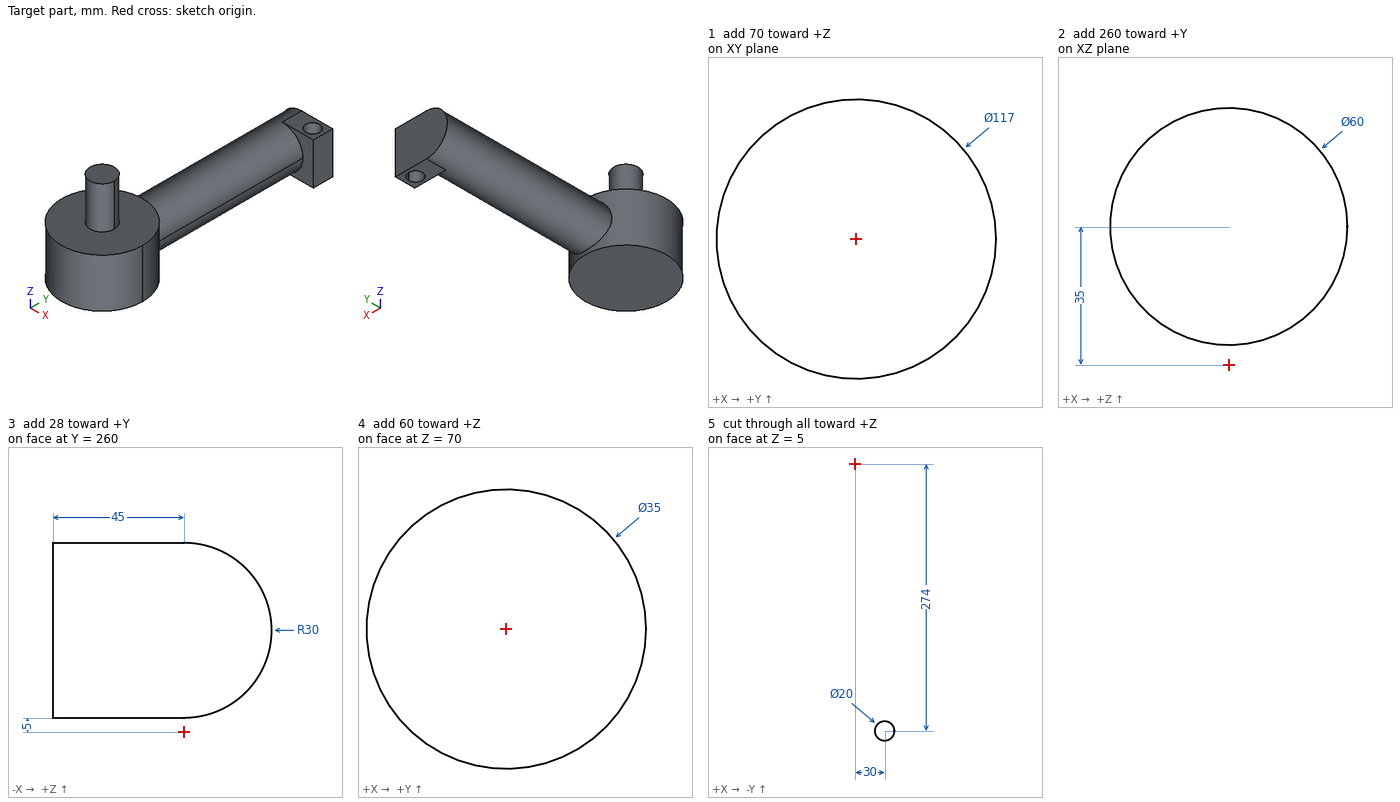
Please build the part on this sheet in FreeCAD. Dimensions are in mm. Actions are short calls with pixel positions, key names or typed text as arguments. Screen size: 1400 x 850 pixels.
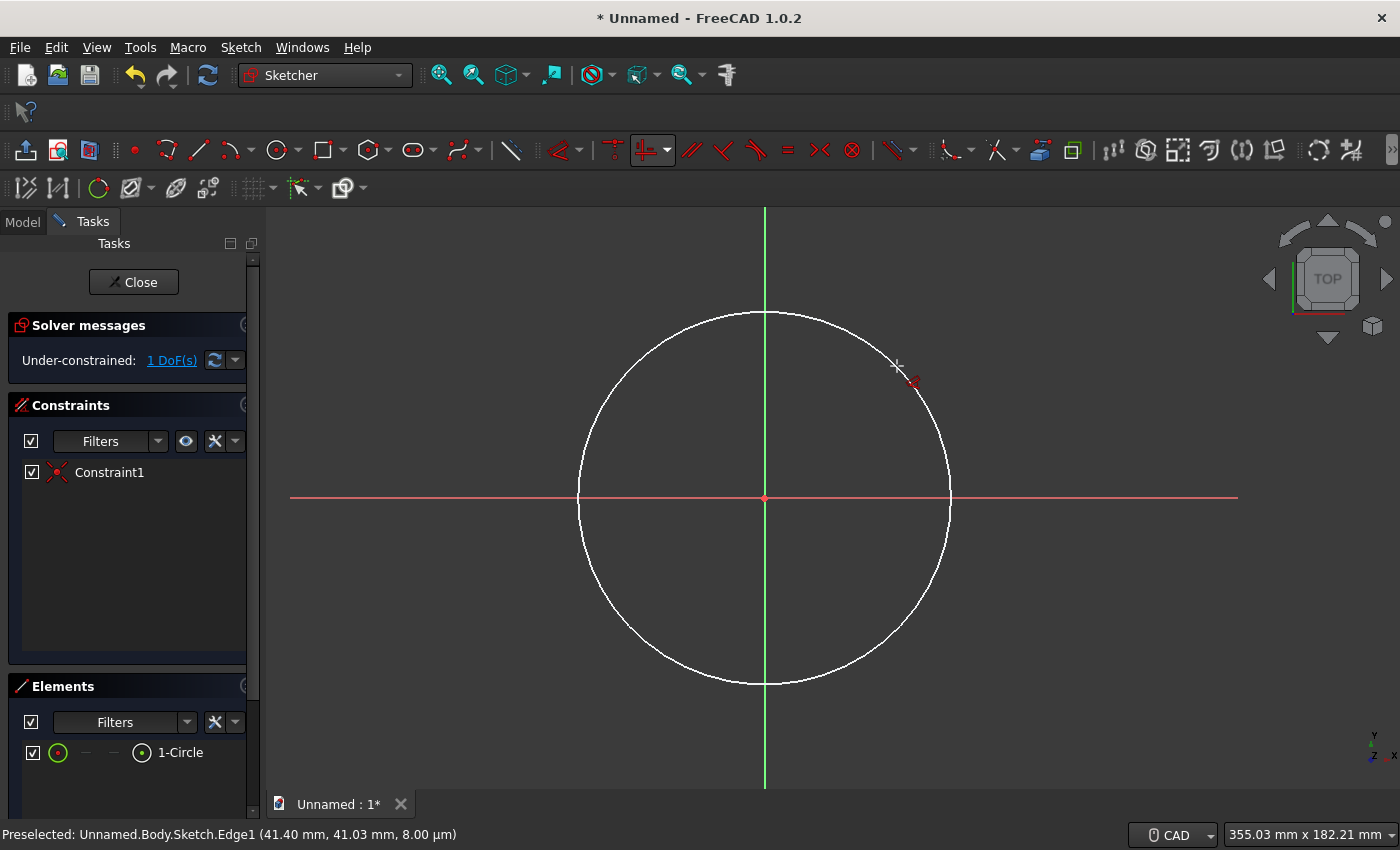
click(896, 366)
click(919, 343)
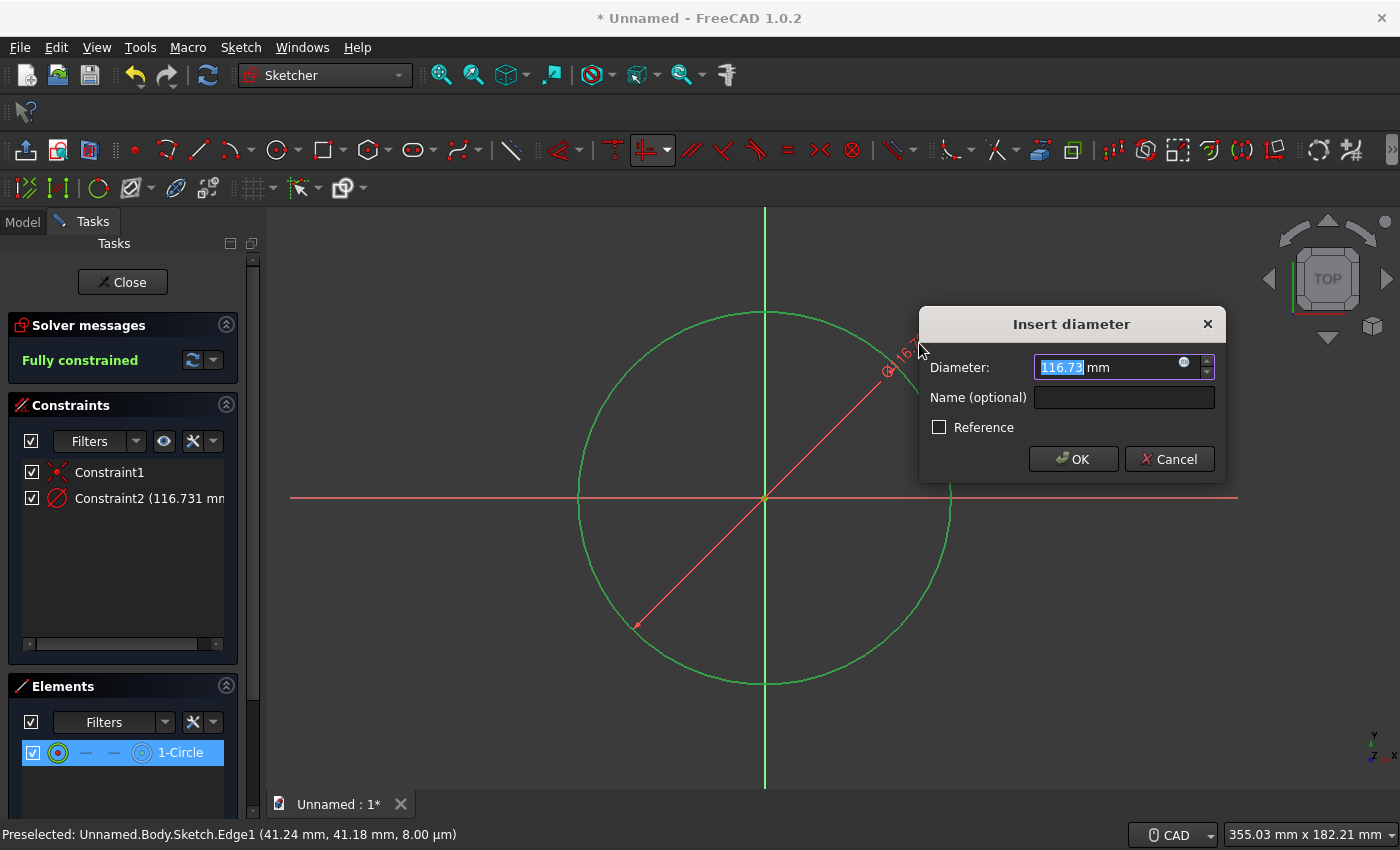
text(117)
key(Return)
key(Escape)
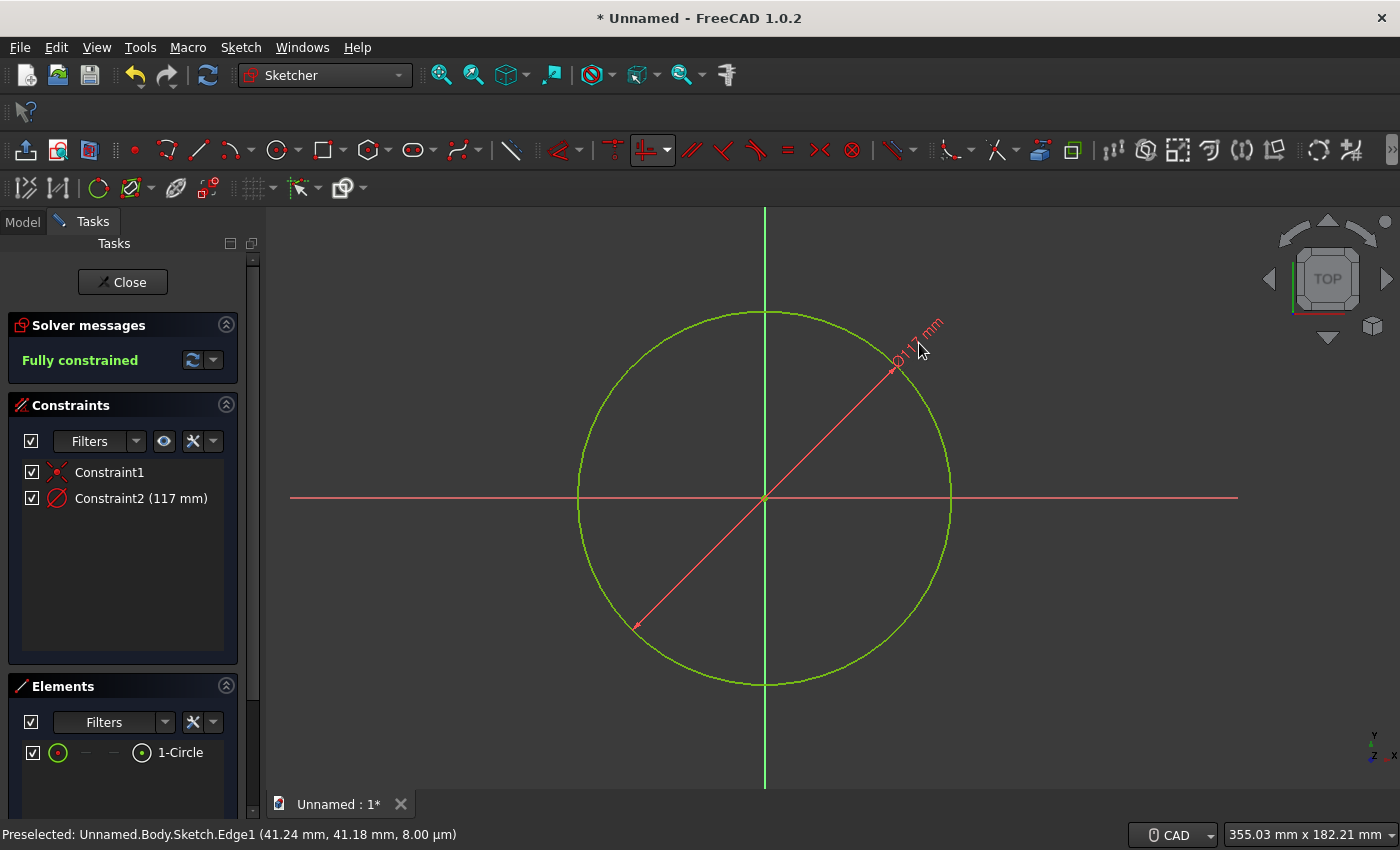
click(123, 282)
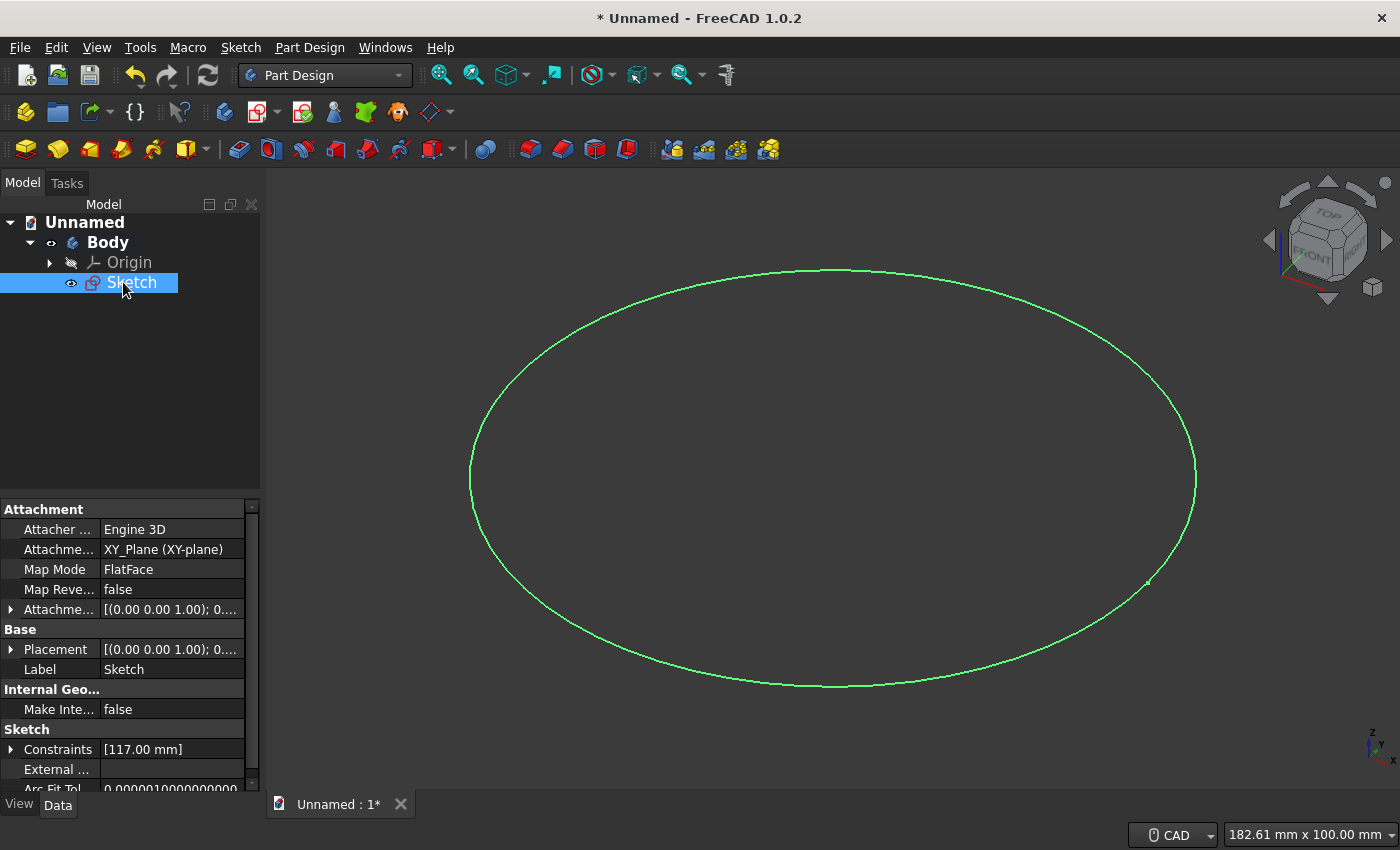
click(26, 150)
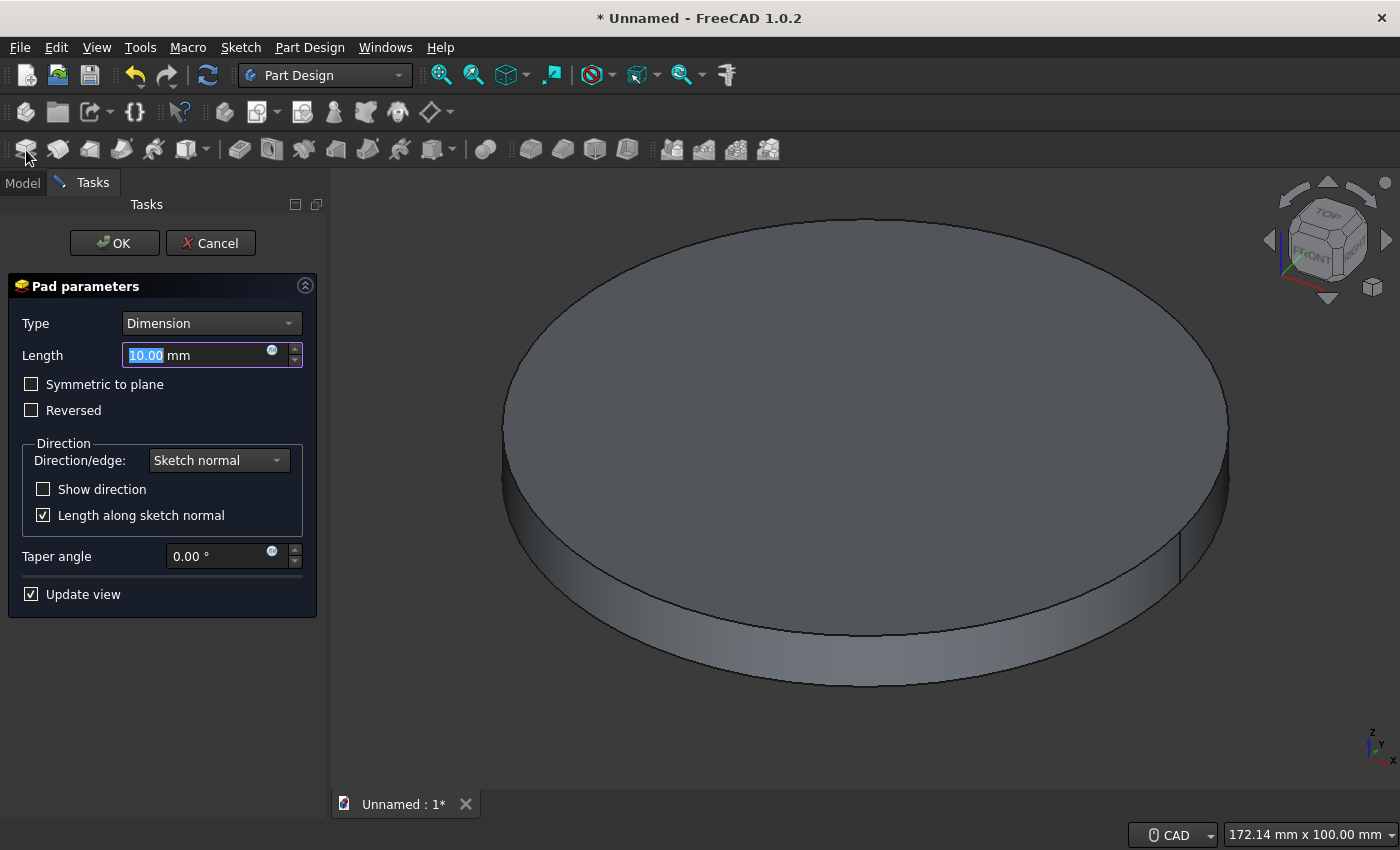
text(70)
key(Tab)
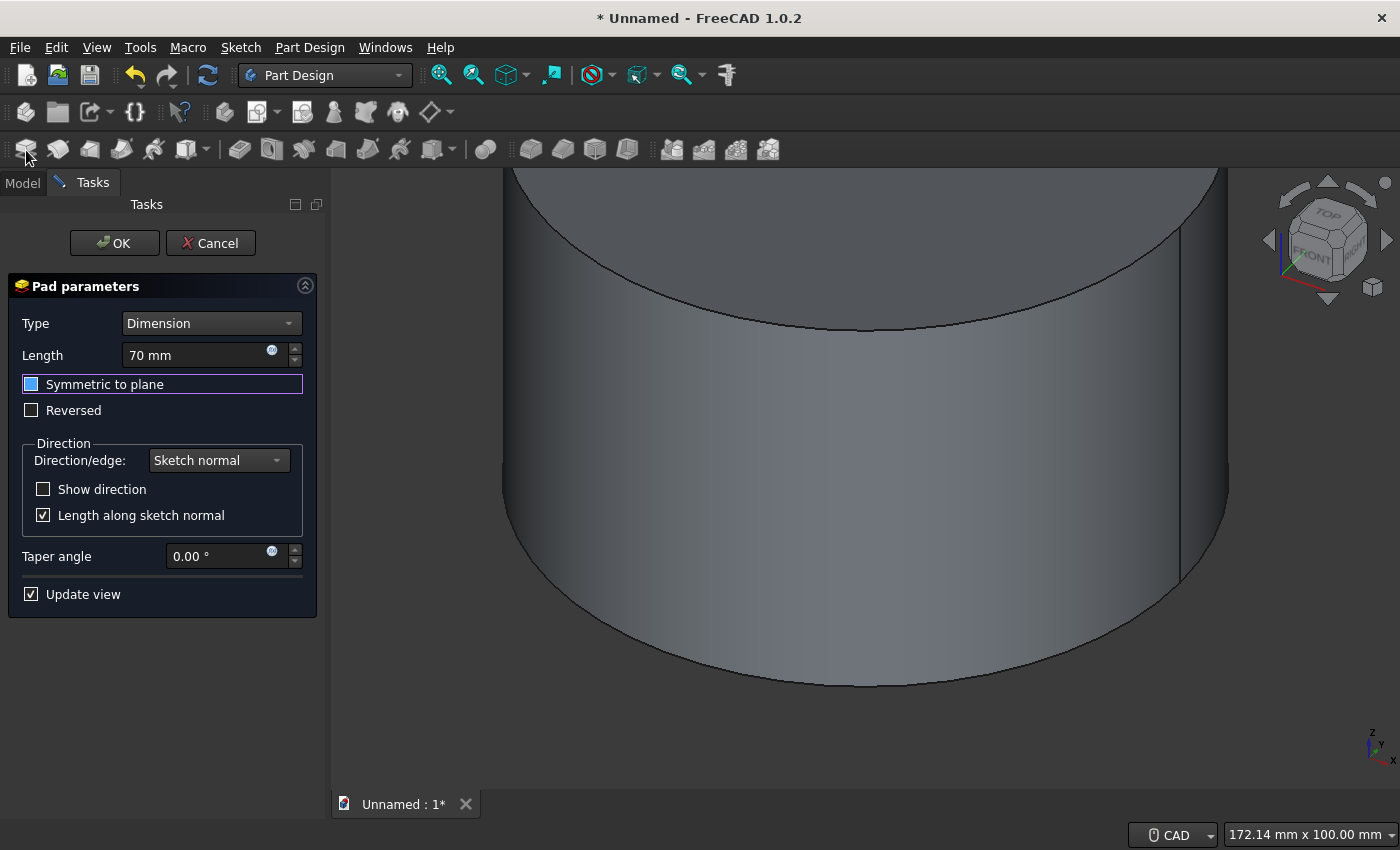
click(115, 243)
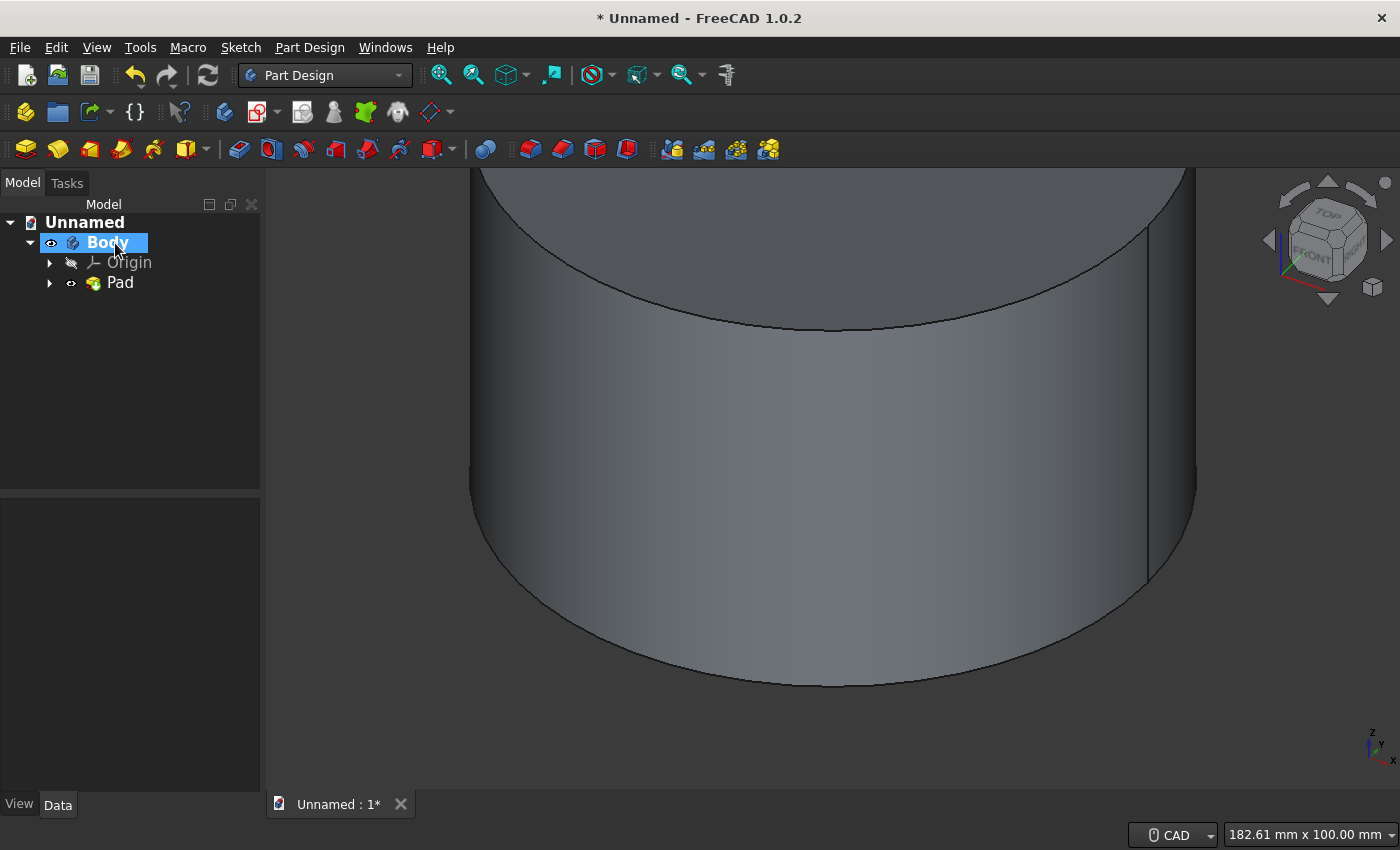
click(442, 76)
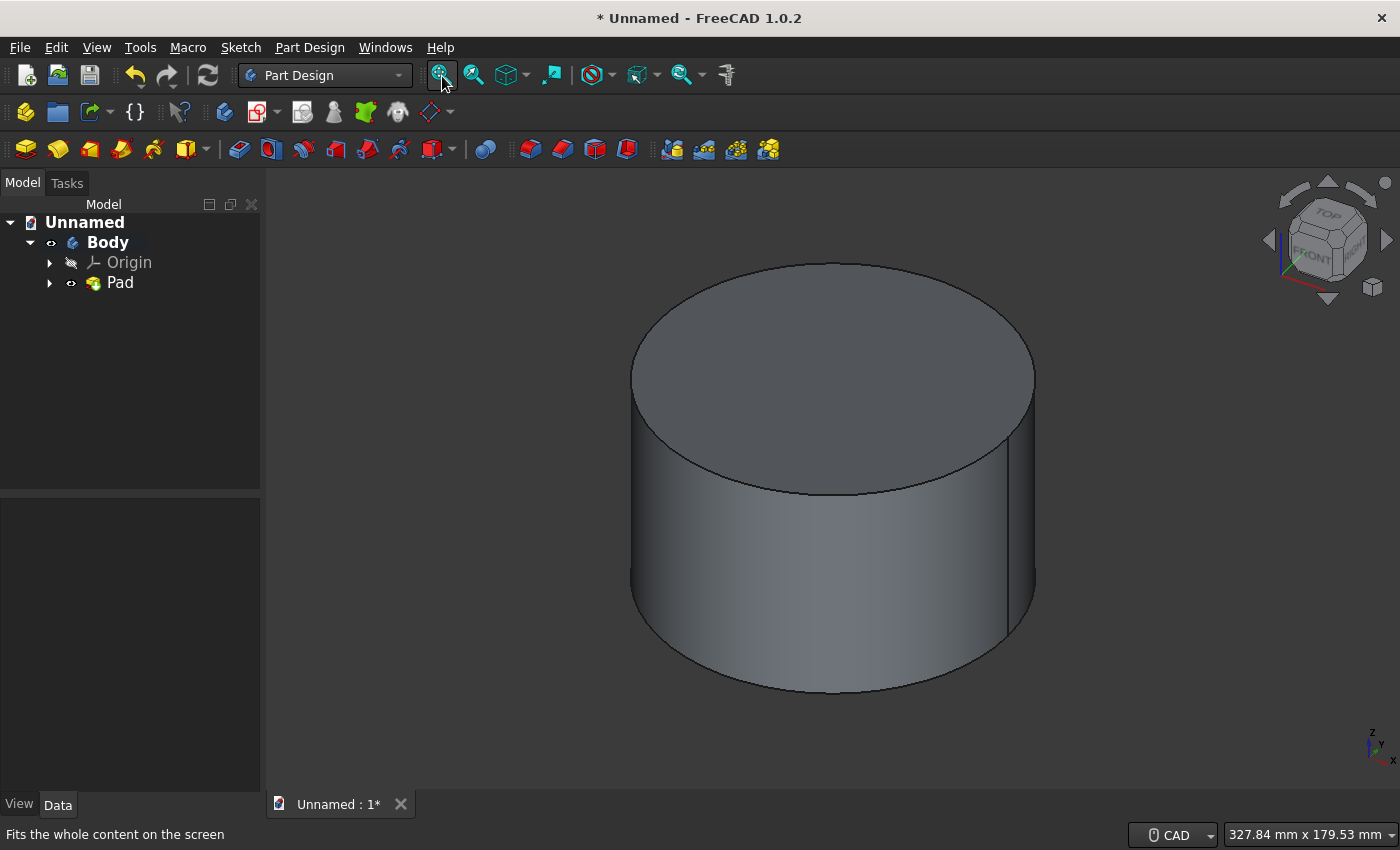
click(258, 112)